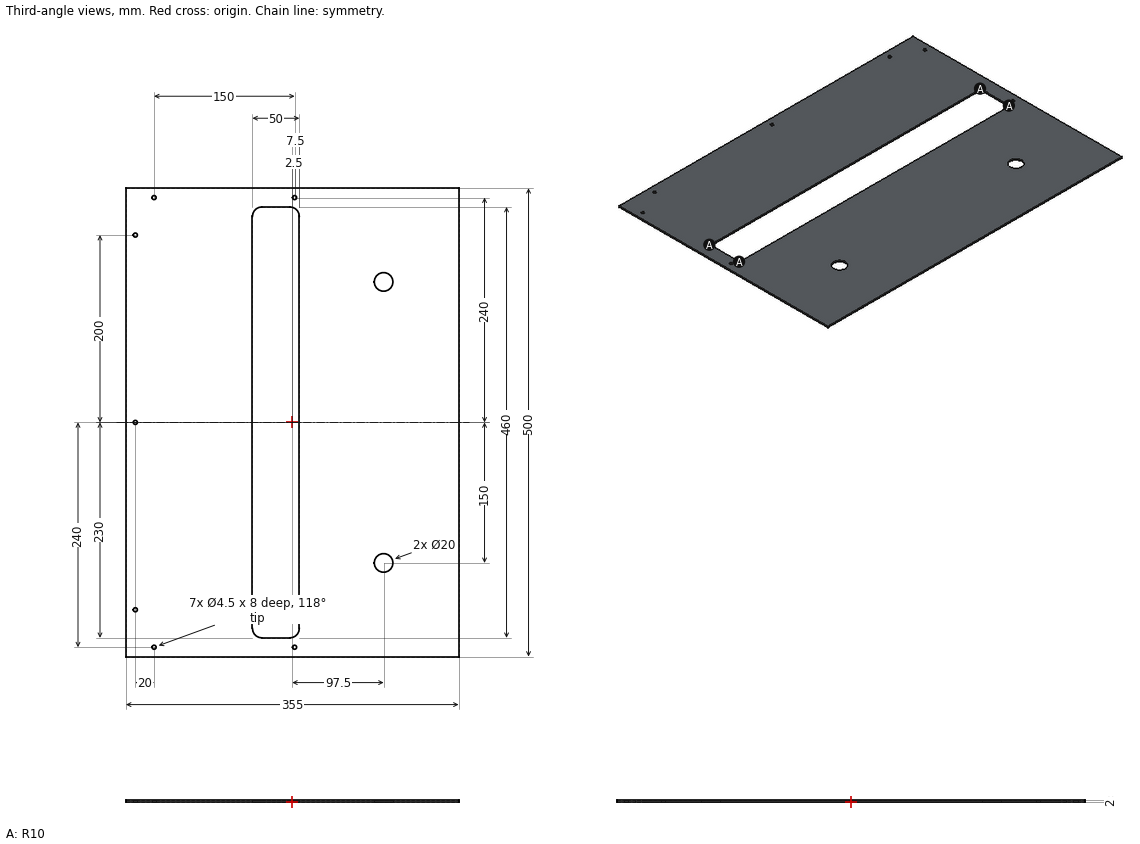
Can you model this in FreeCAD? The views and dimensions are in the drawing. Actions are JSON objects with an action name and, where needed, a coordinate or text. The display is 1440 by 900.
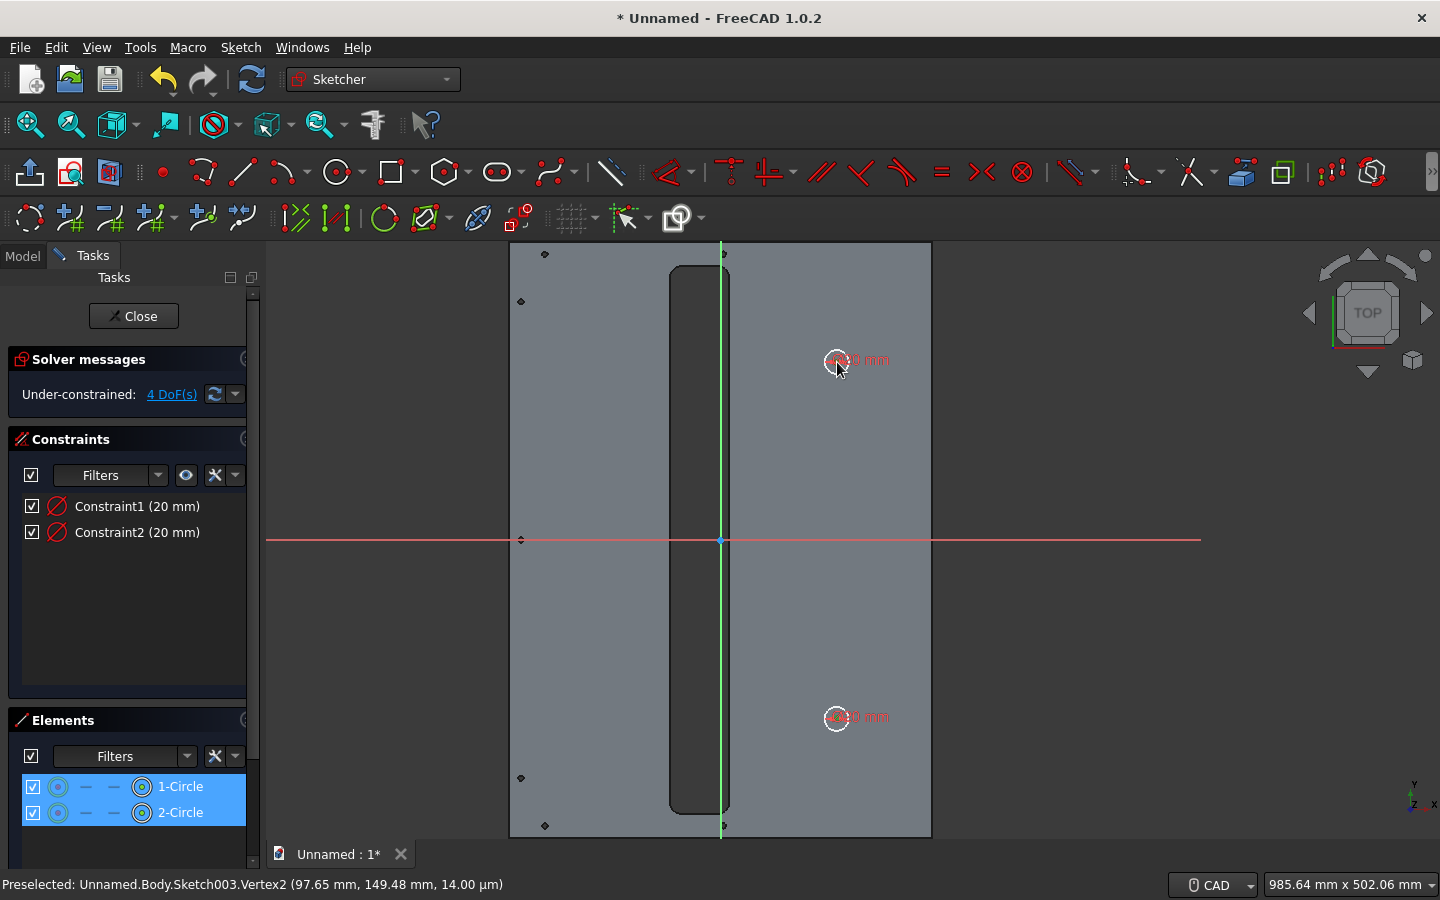
{"action": "left_click", "coordinate": [364, 540]}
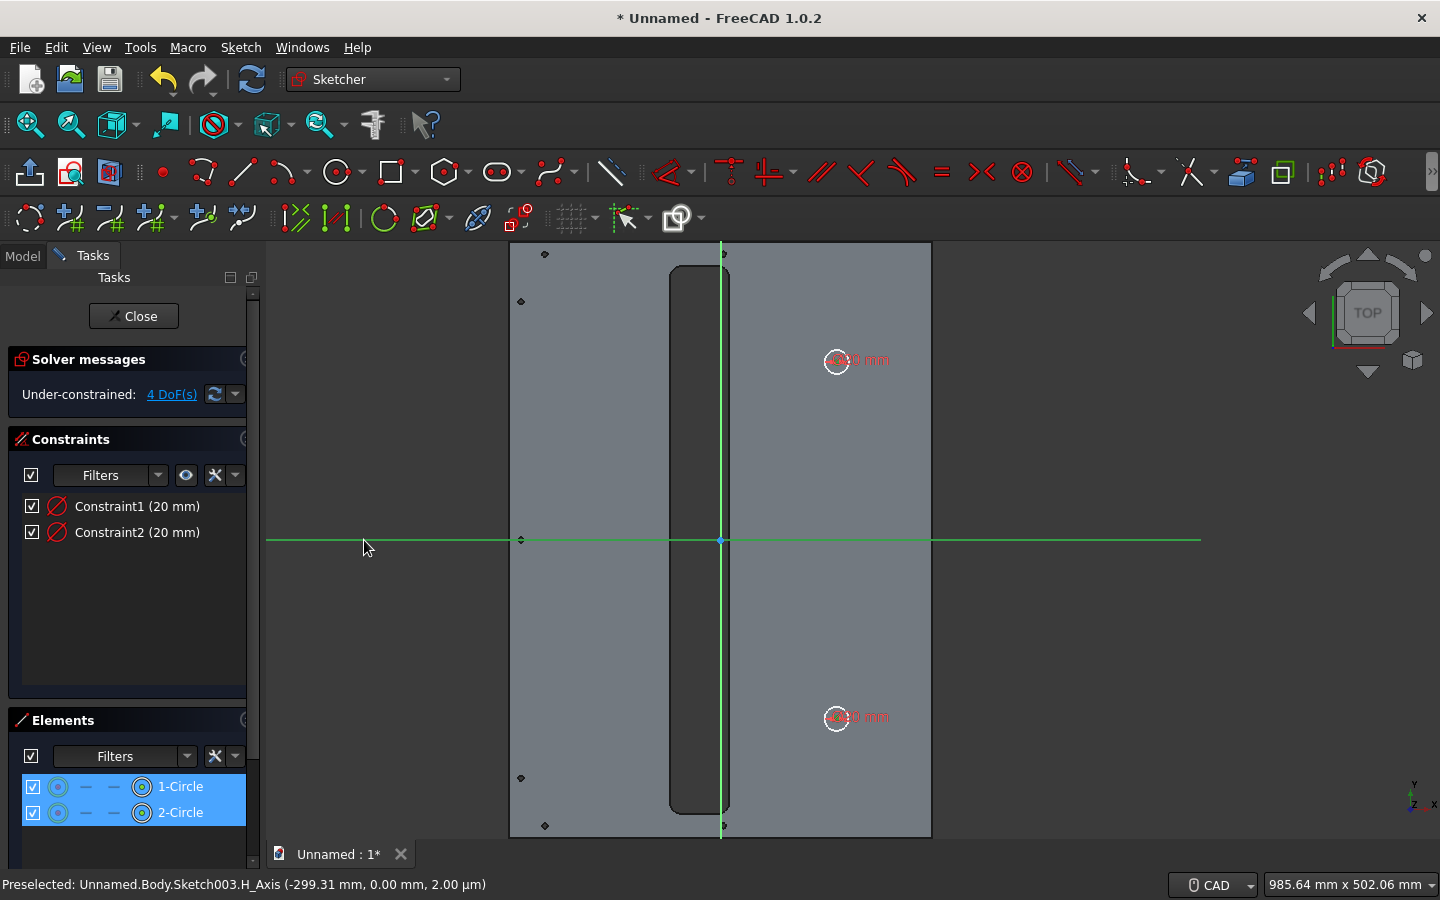
{"action": "left_click", "coordinate": [982, 172]}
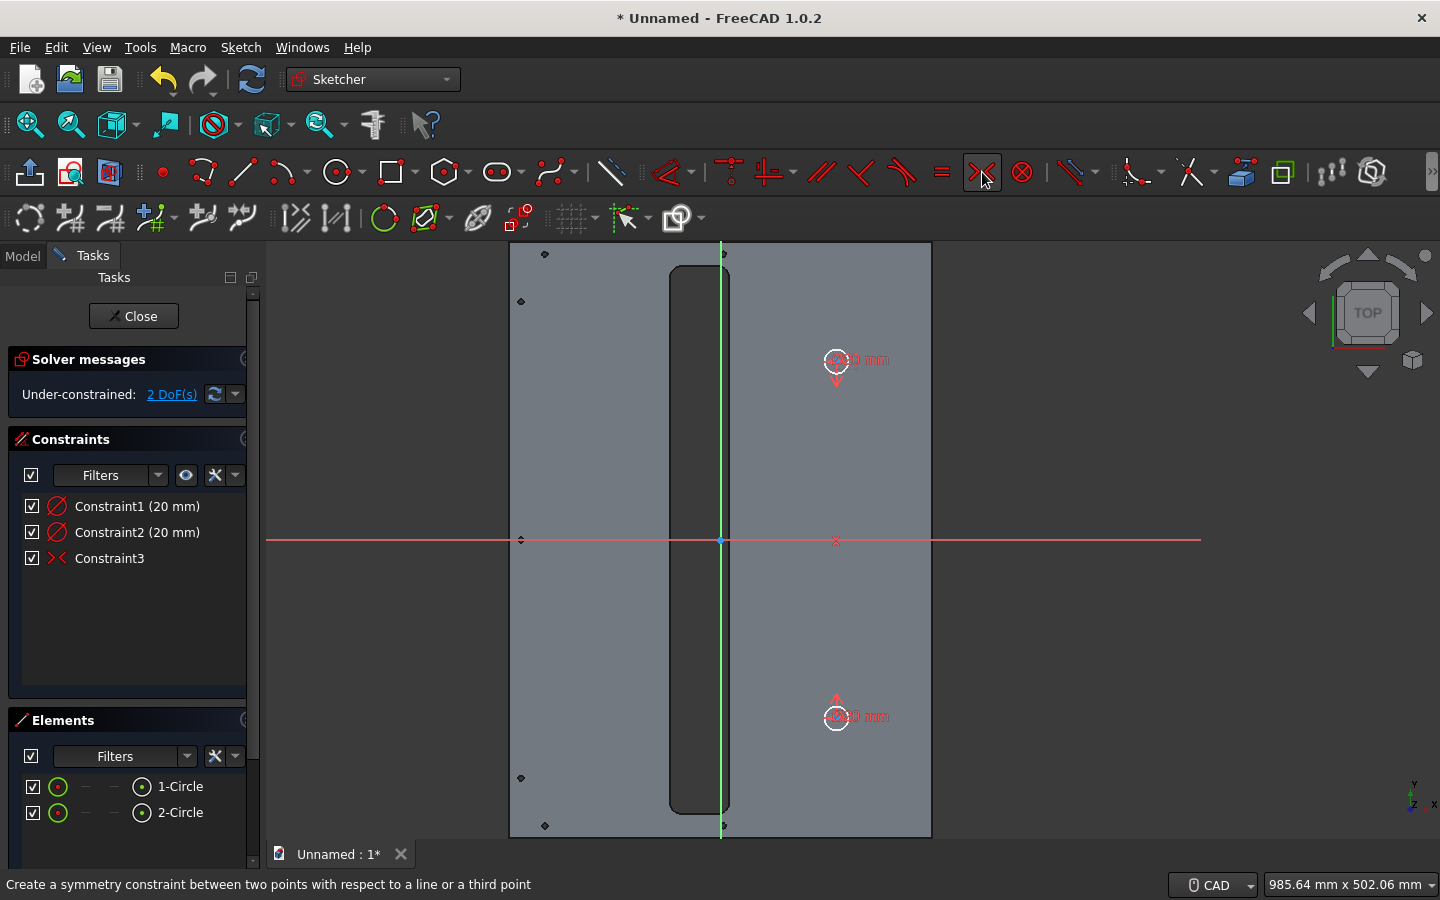
{"action": "left_click", "coordinate": [666, 172]}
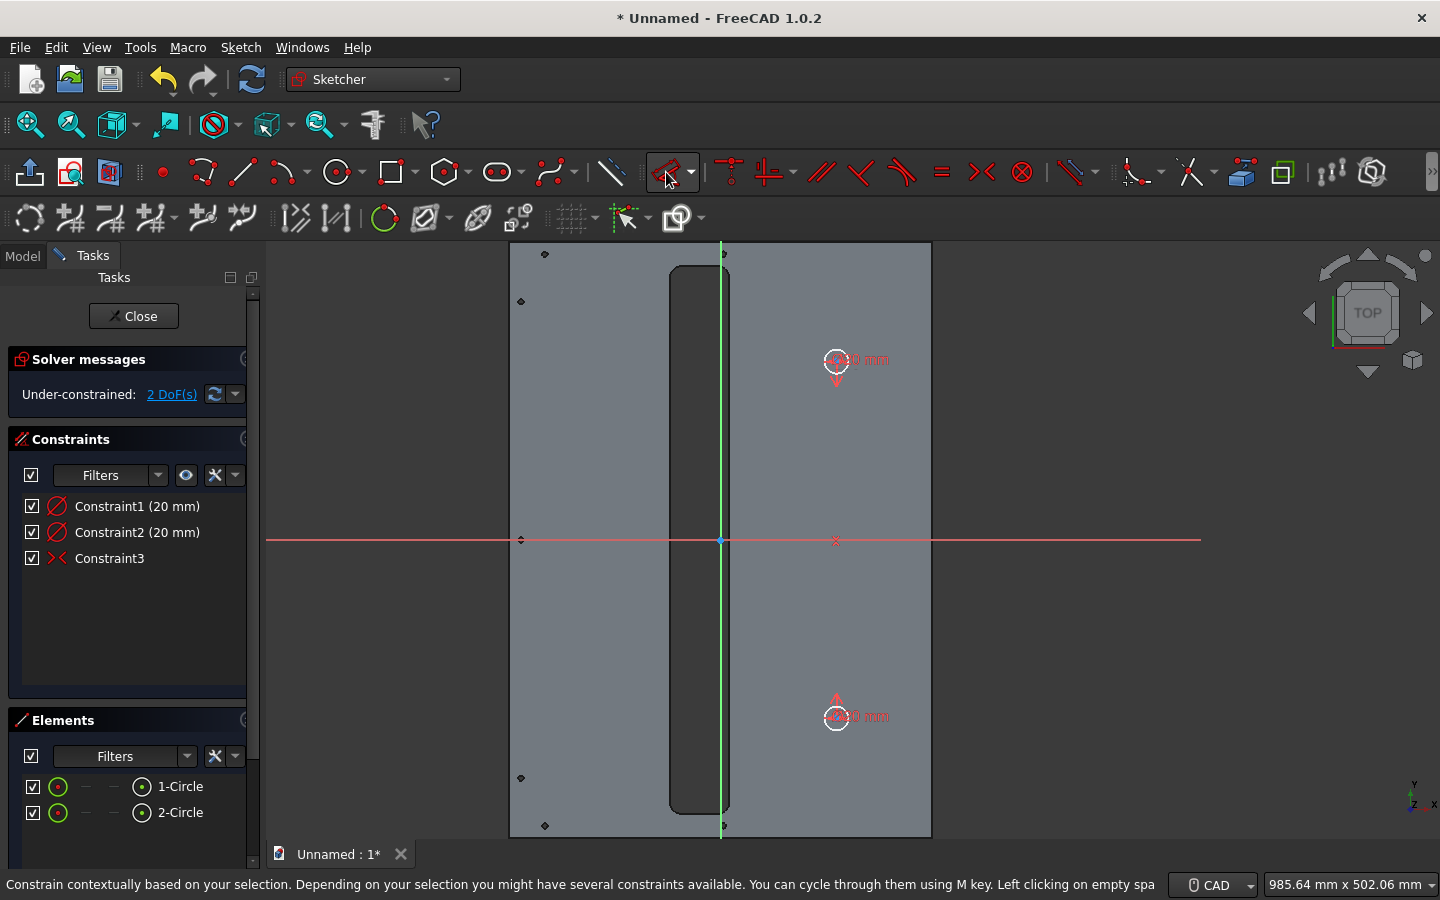
{"action": "left_click", "coordinate": [837, 718]}
{"action": "left_click", "coordinate": [687, 629]}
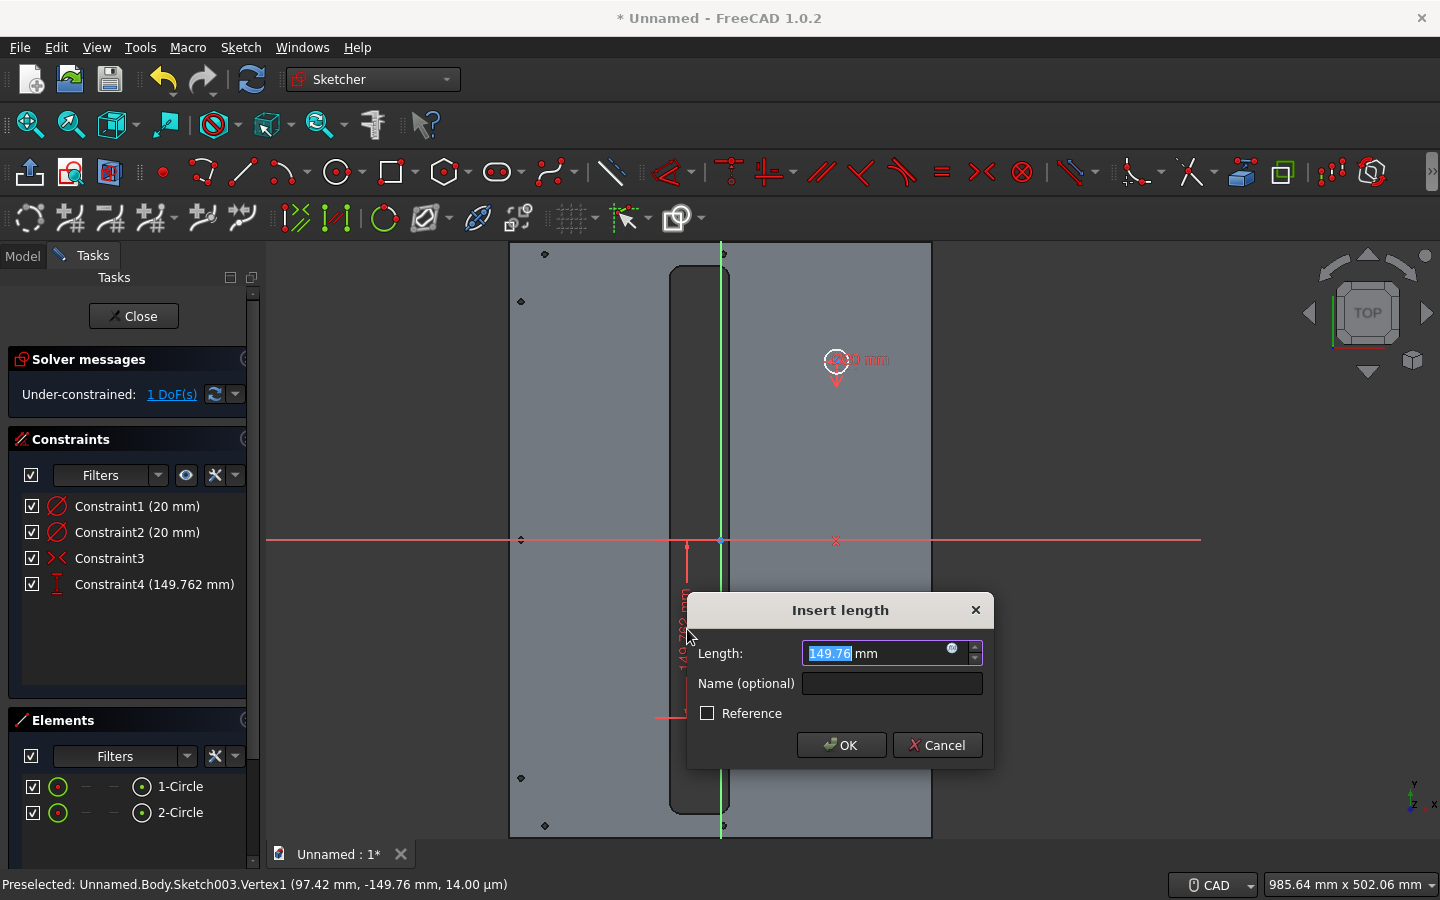
{"action": "type", "text": "150"}
{"action": "key", "text": "Return"}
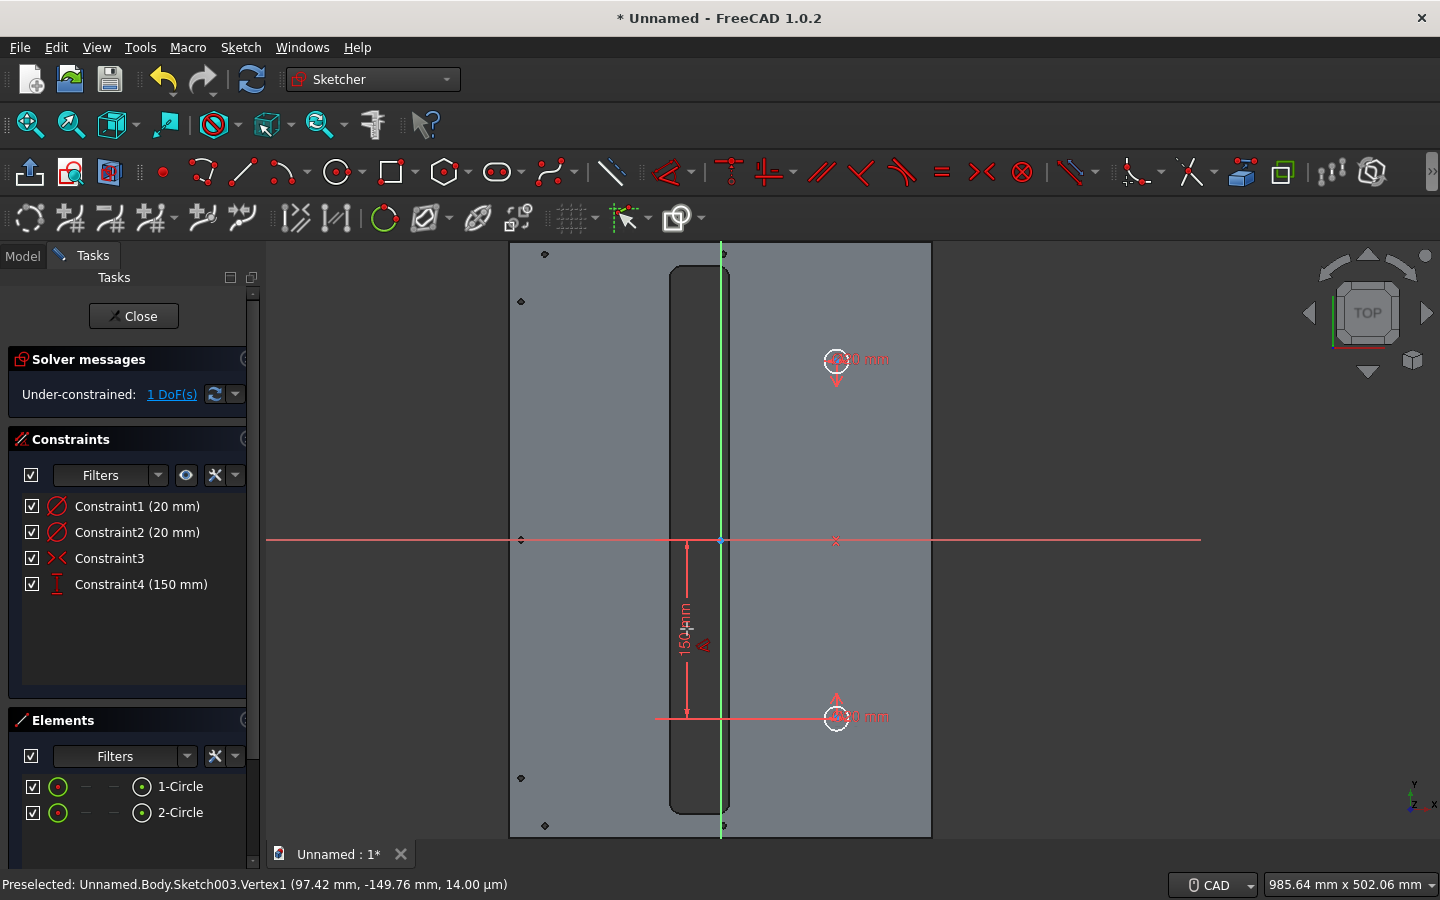
{"action": "left_click", "coordinate": [837, 719]}
{"action": "left_click", "coordinate": [779, 753]}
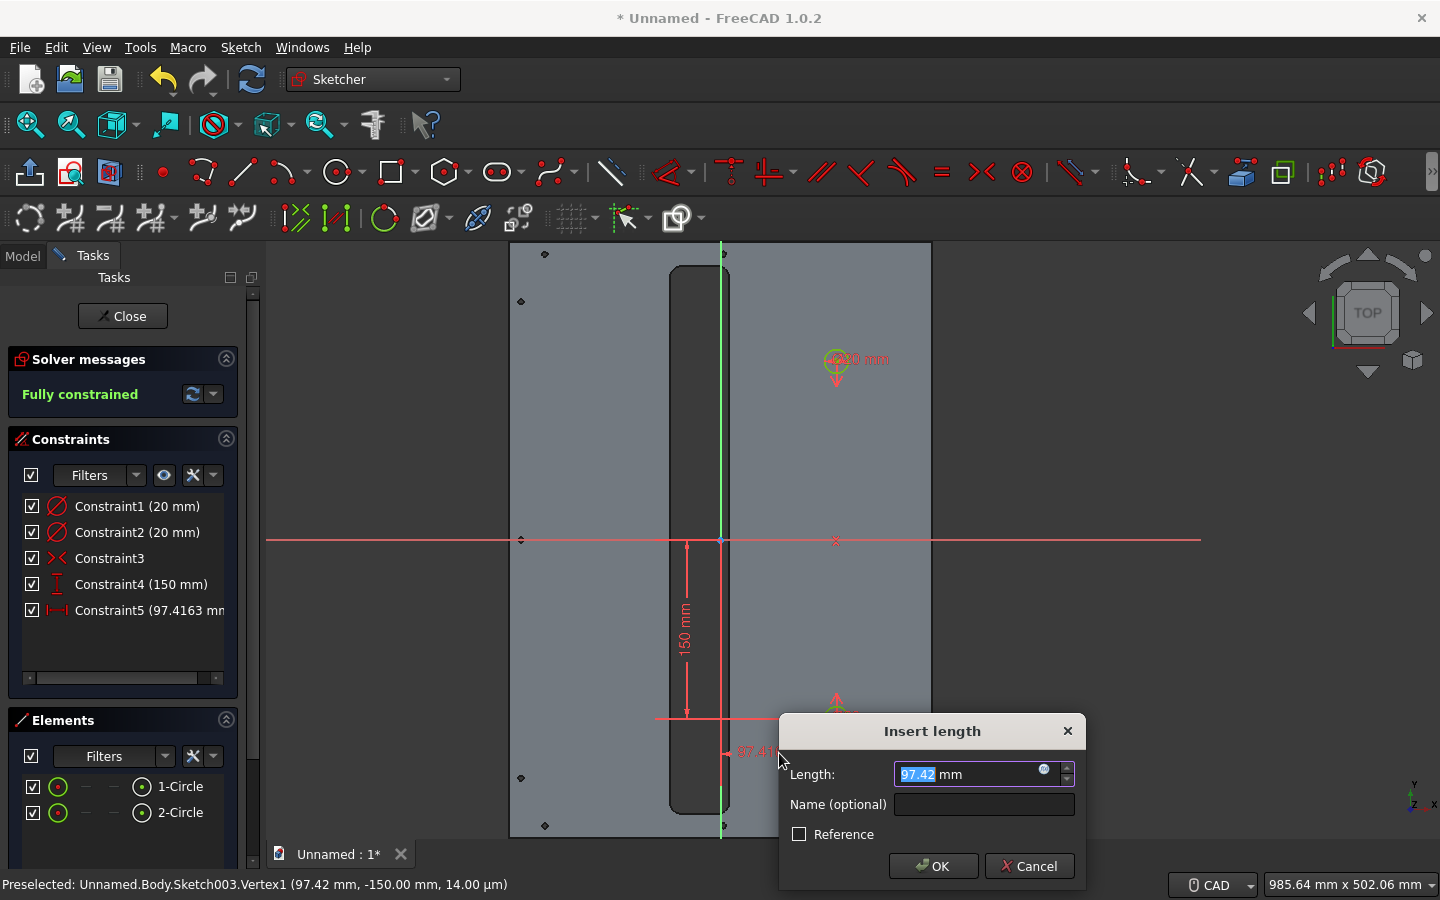
{"action": "type", "text": "97.5"}
{"action": "key", "text": "Return"}
{"action": "key", "text": "Escape"}